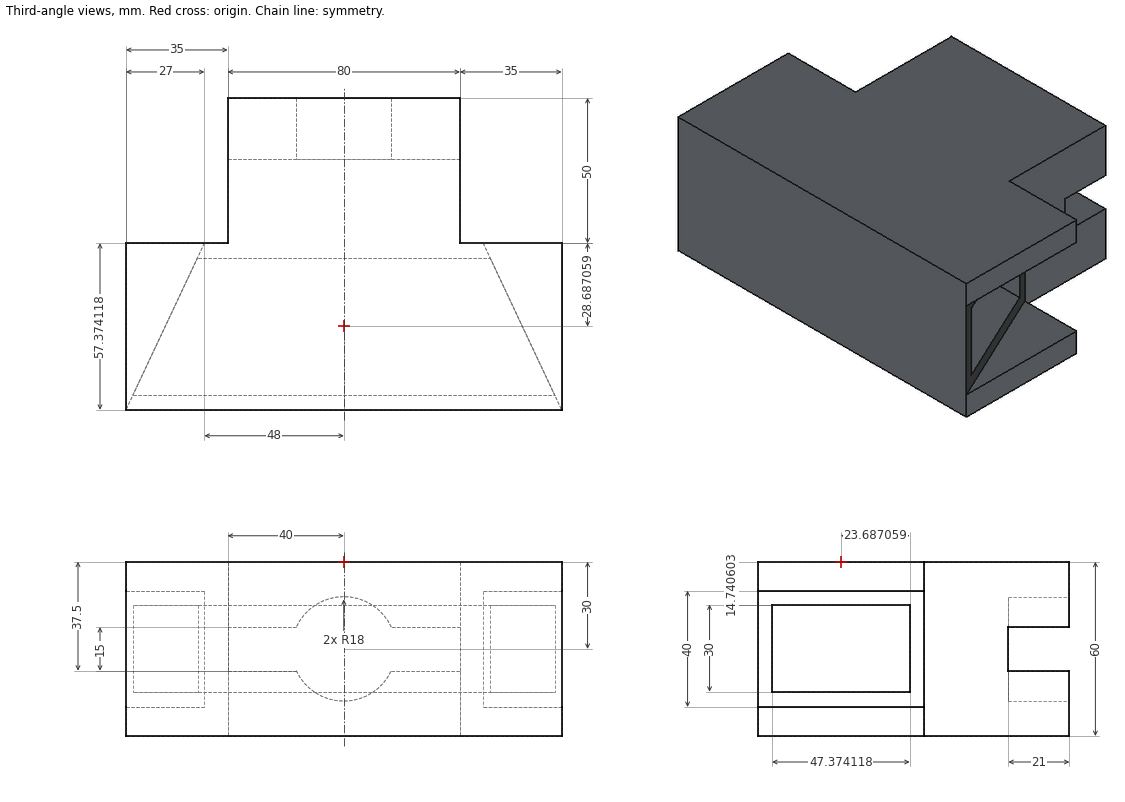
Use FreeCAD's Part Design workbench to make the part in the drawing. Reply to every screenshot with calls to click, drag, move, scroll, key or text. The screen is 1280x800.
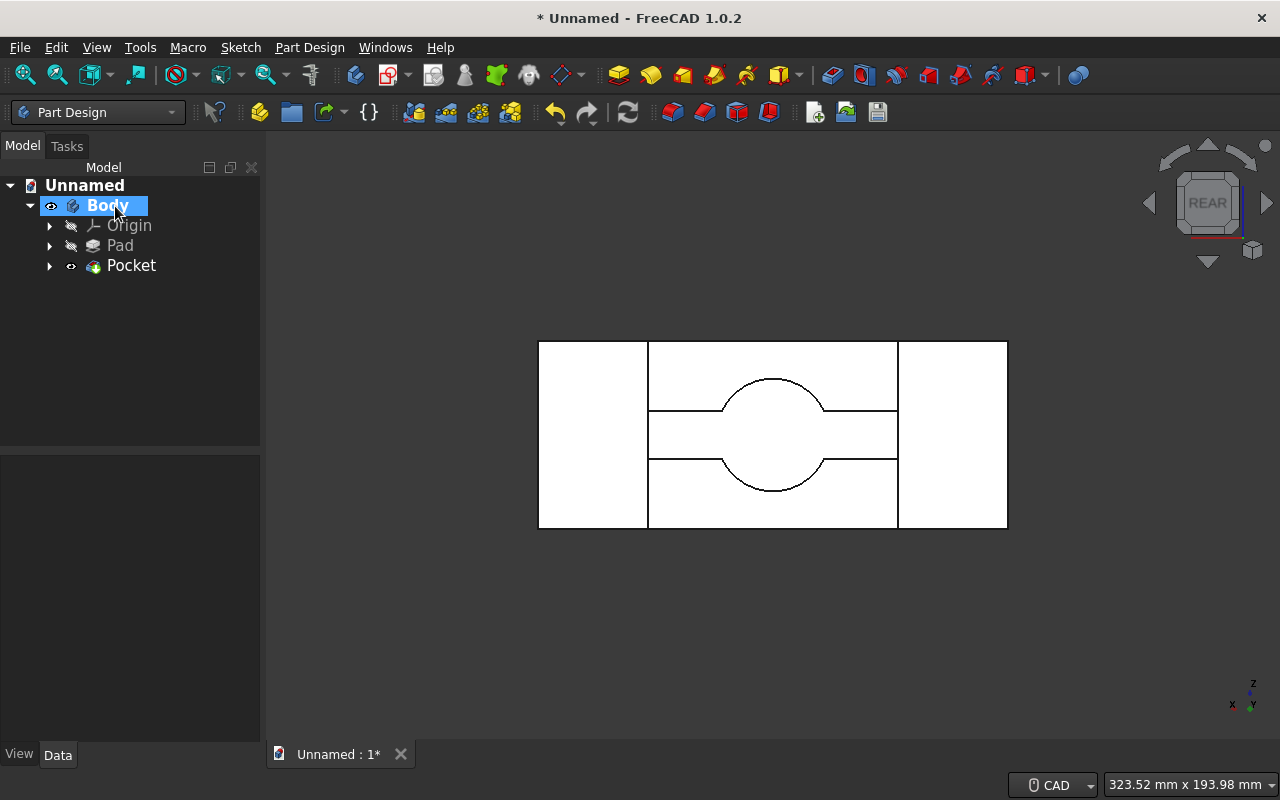
key(6)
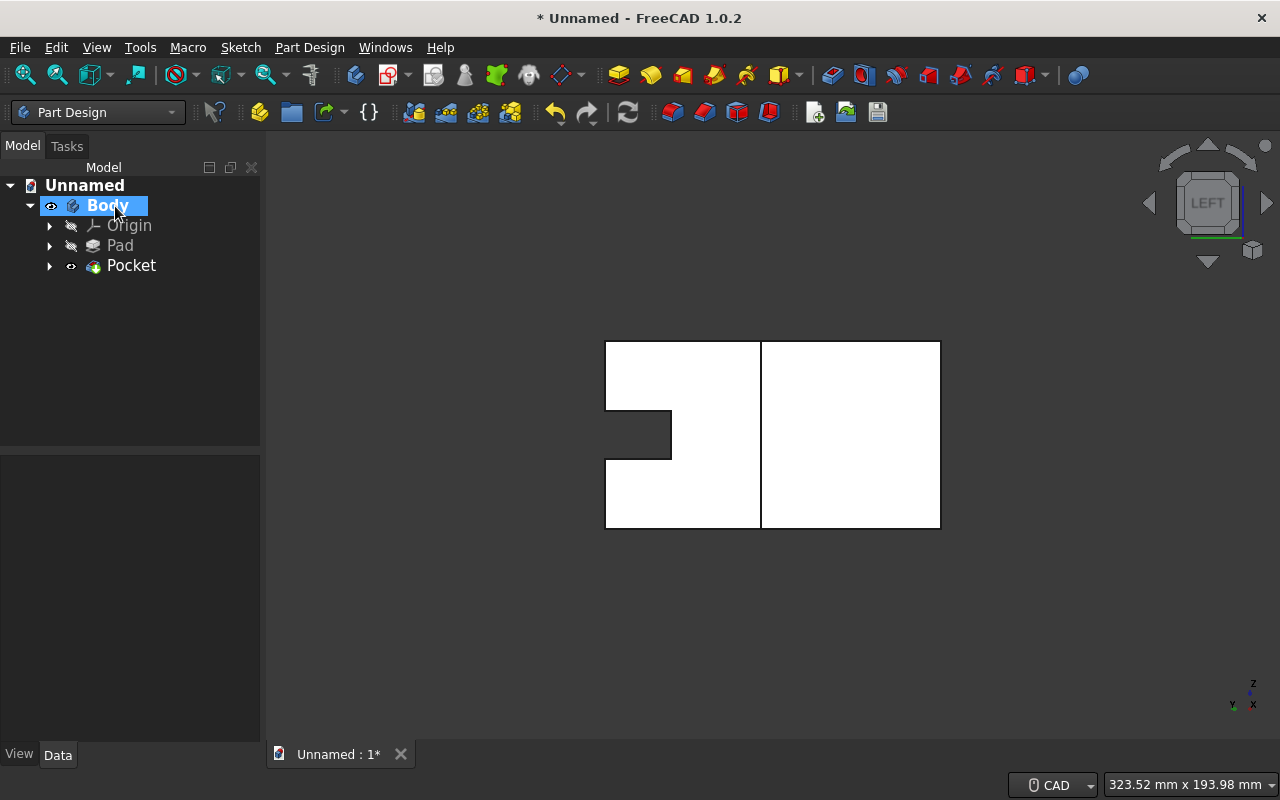
key(v)
key(f)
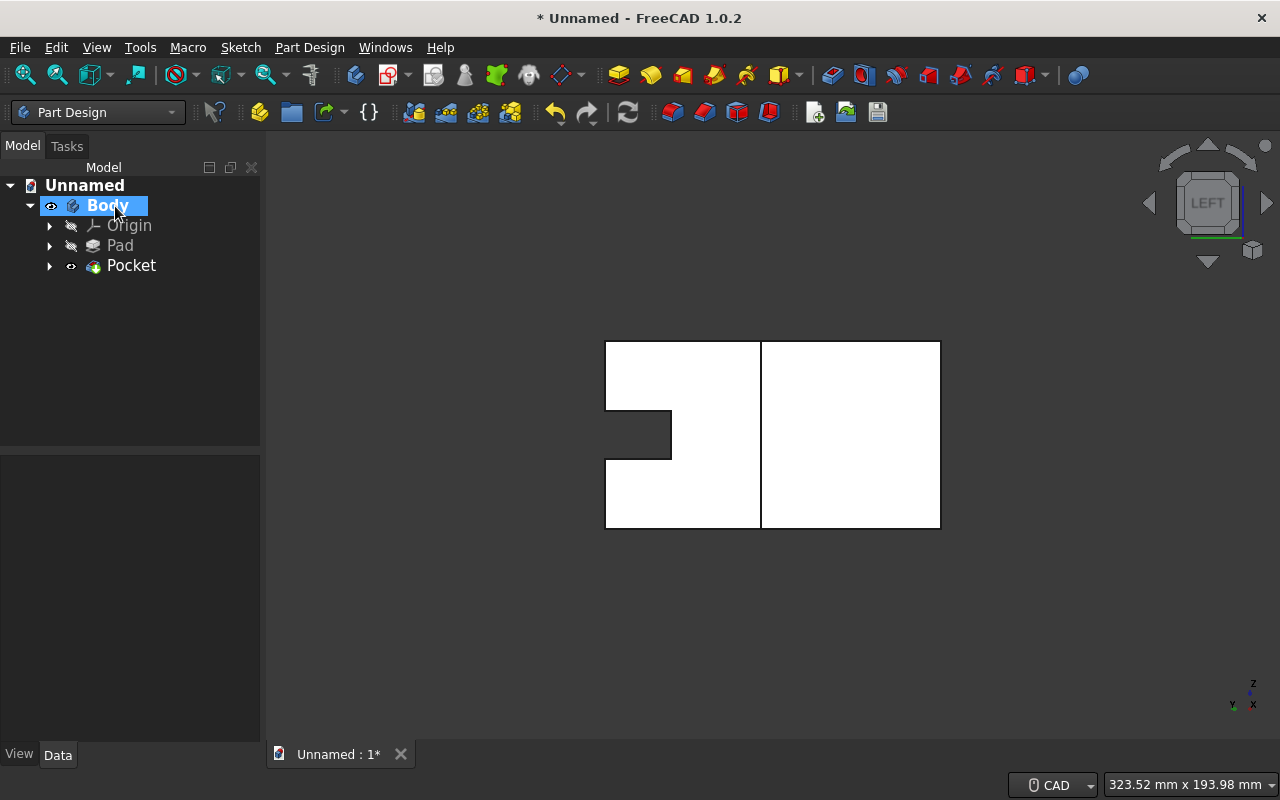
click(851, 434)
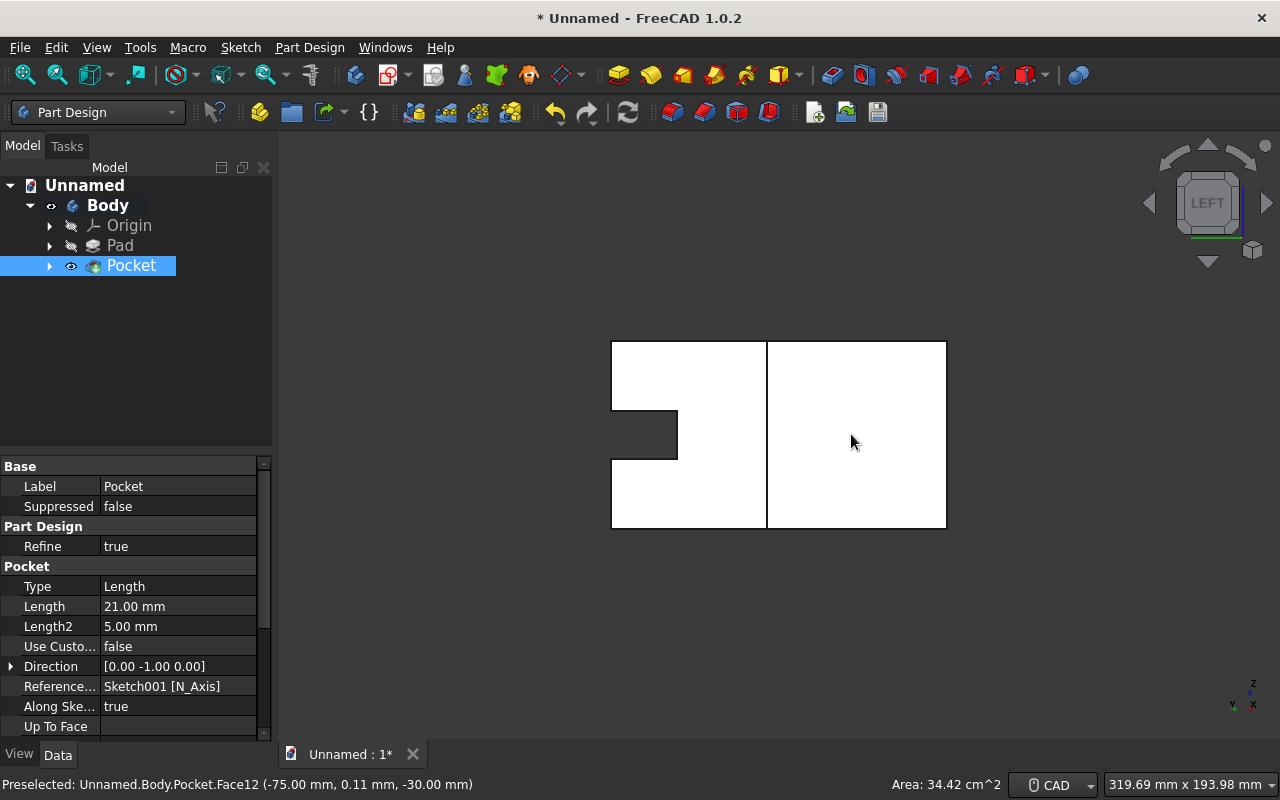
click(388, 76)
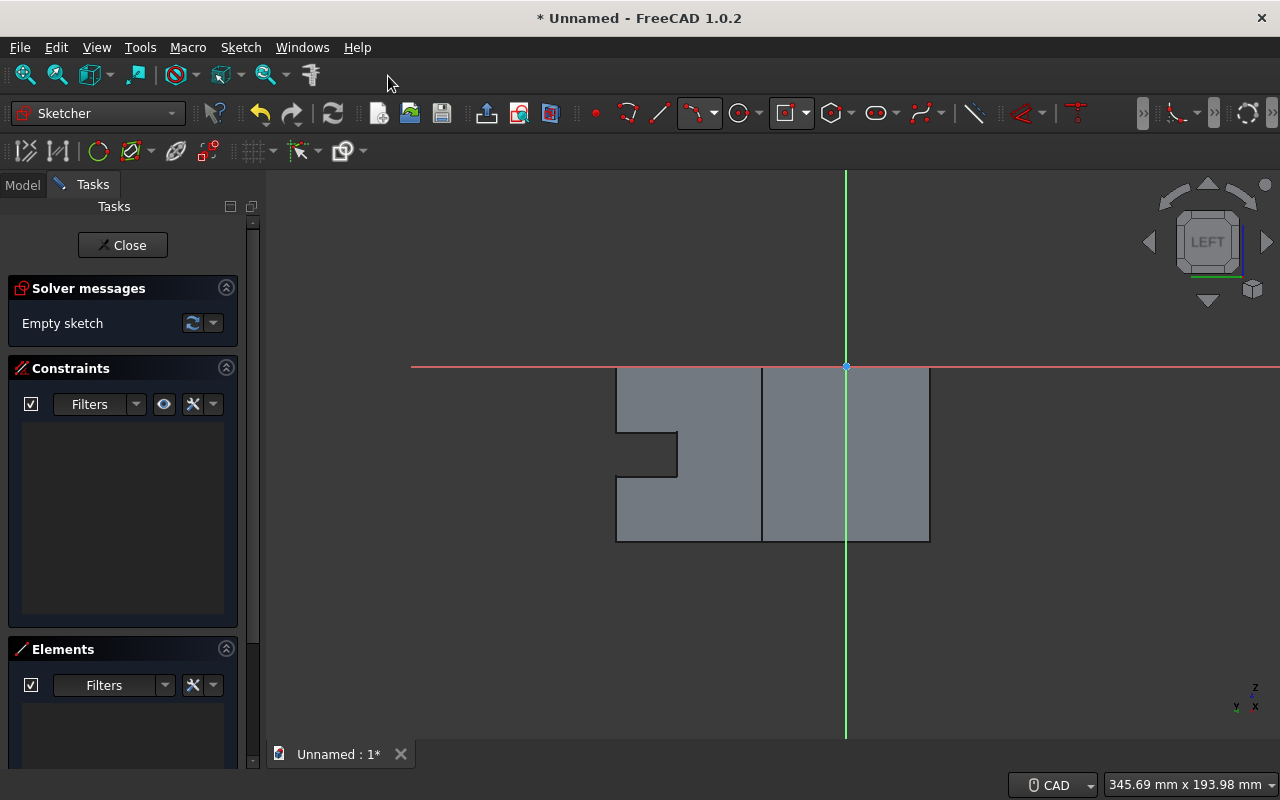
scroll(929, 419, up, 5)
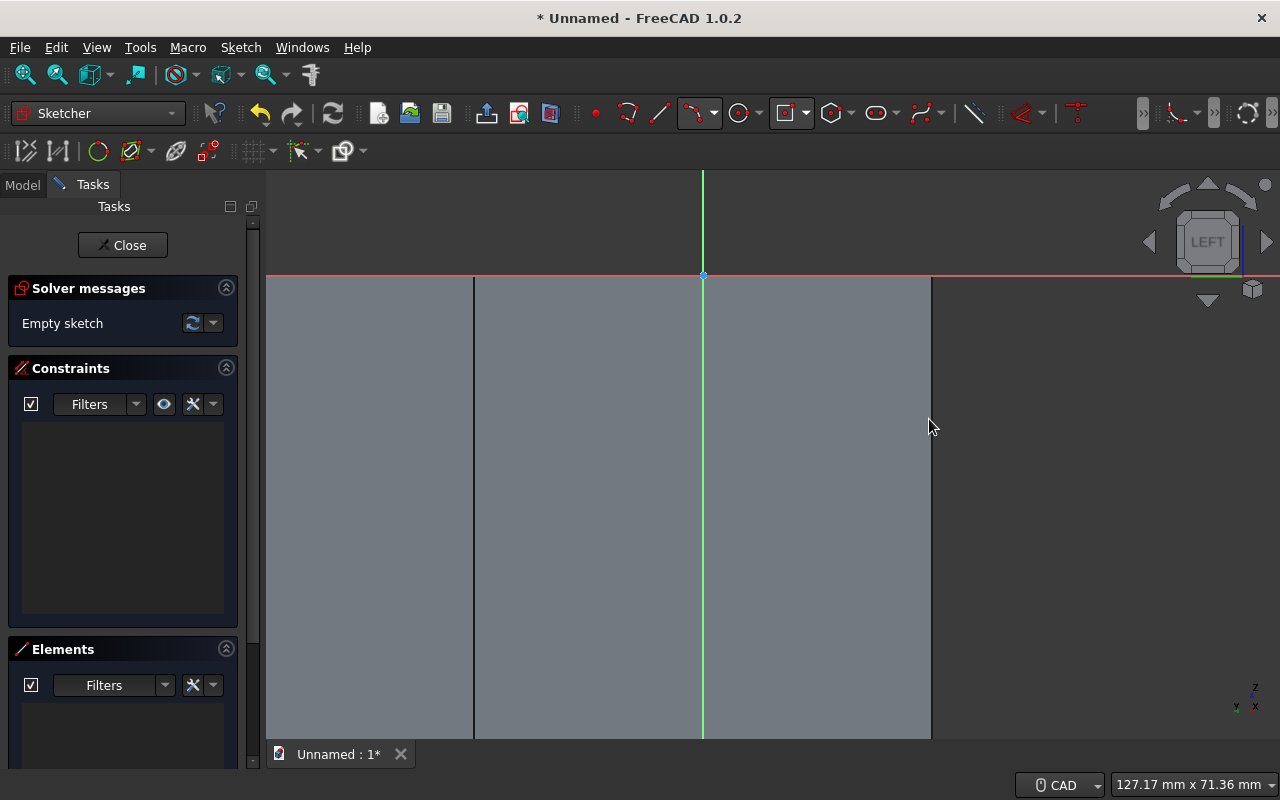
key(g)
key(r)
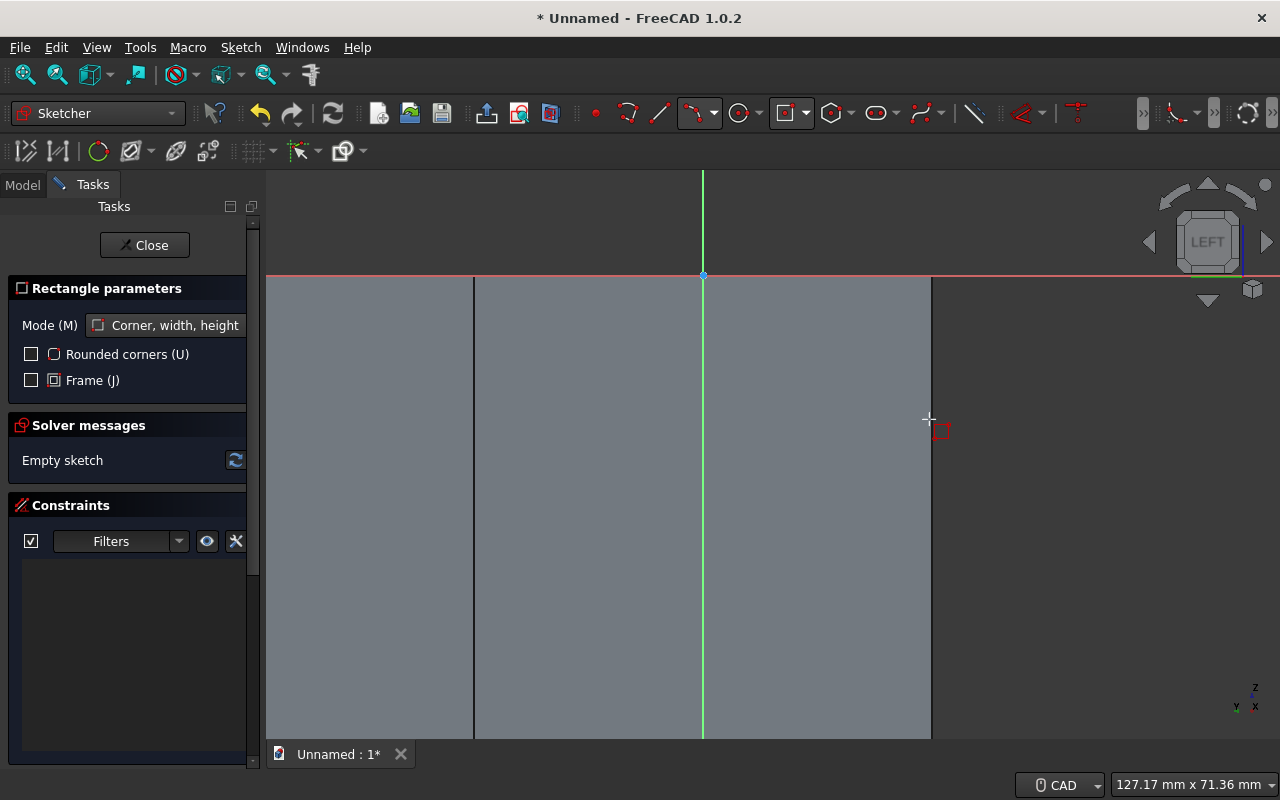
click(514, 393)
move(892, 632)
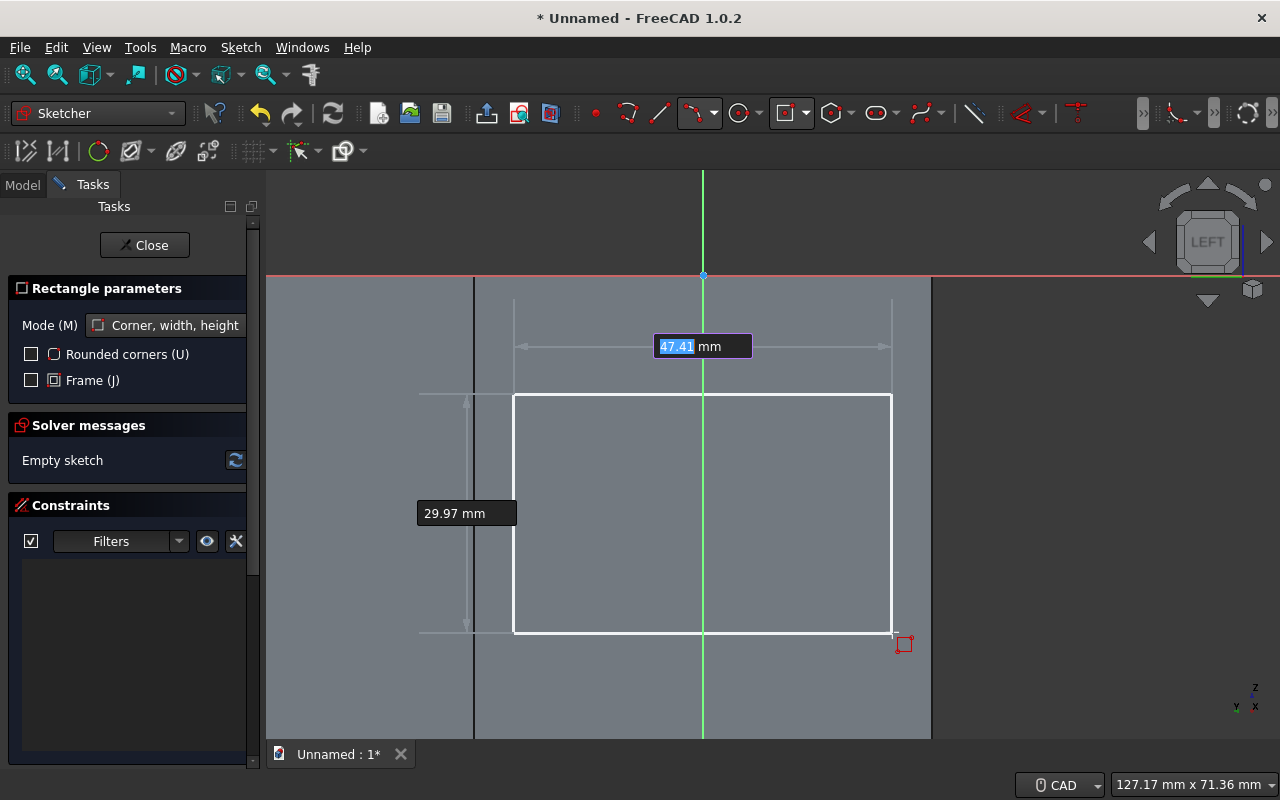
text(47.374118)
key(Tab)
text(30)
key(Return)
key(Escape)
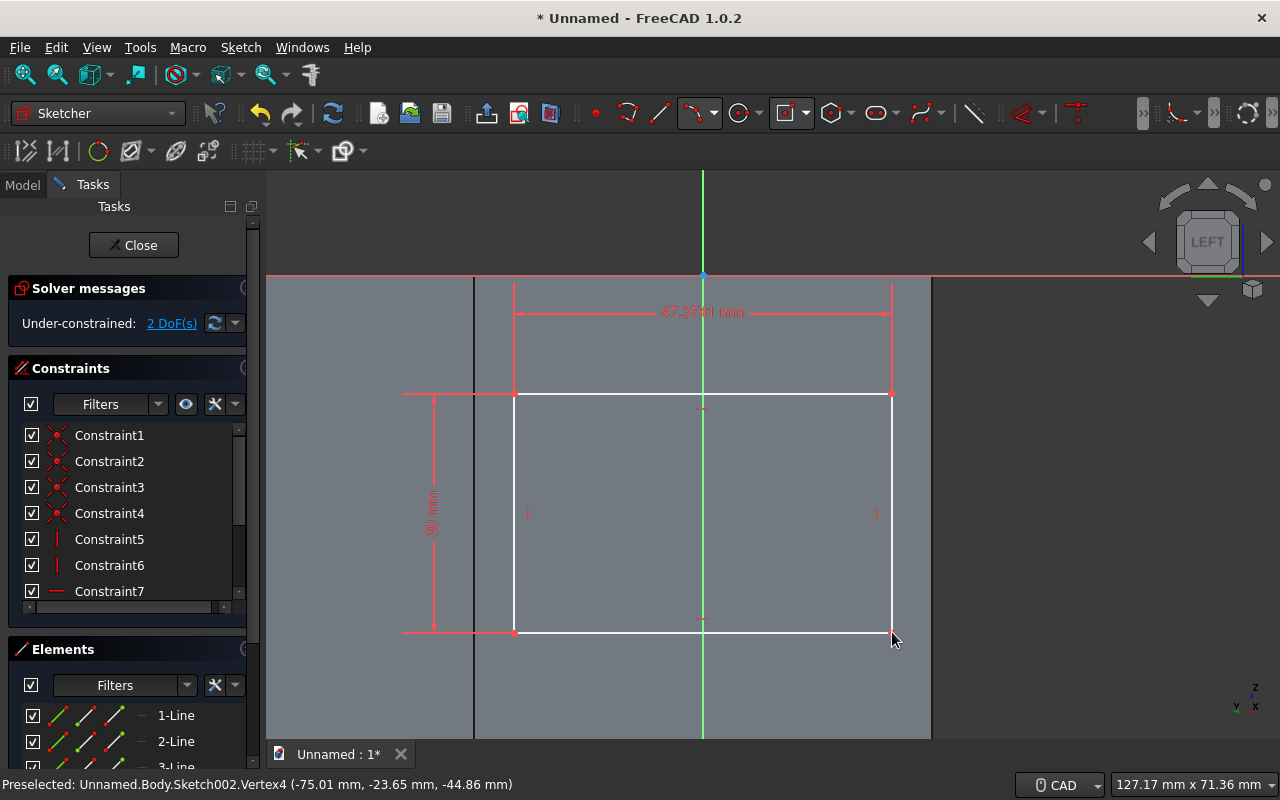
click(1022, 114)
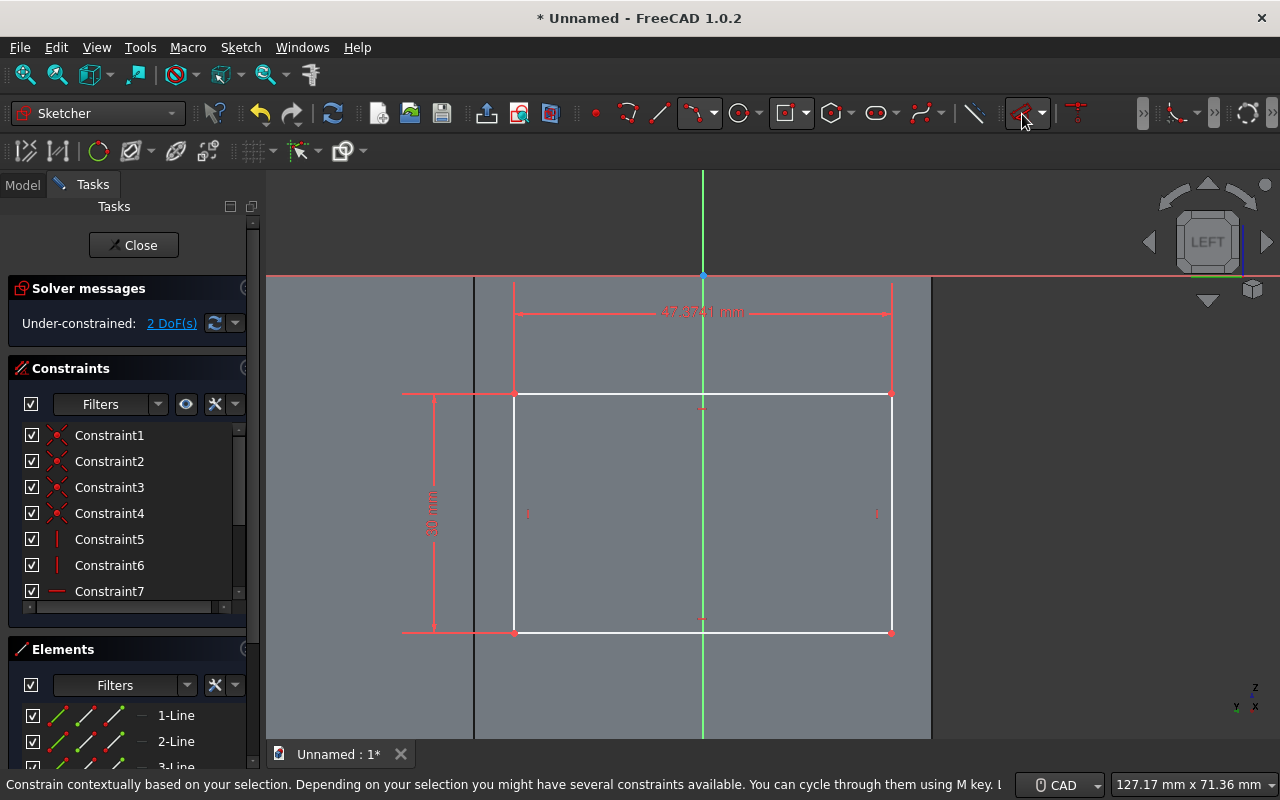
click(514, 394)
click(609, 242)